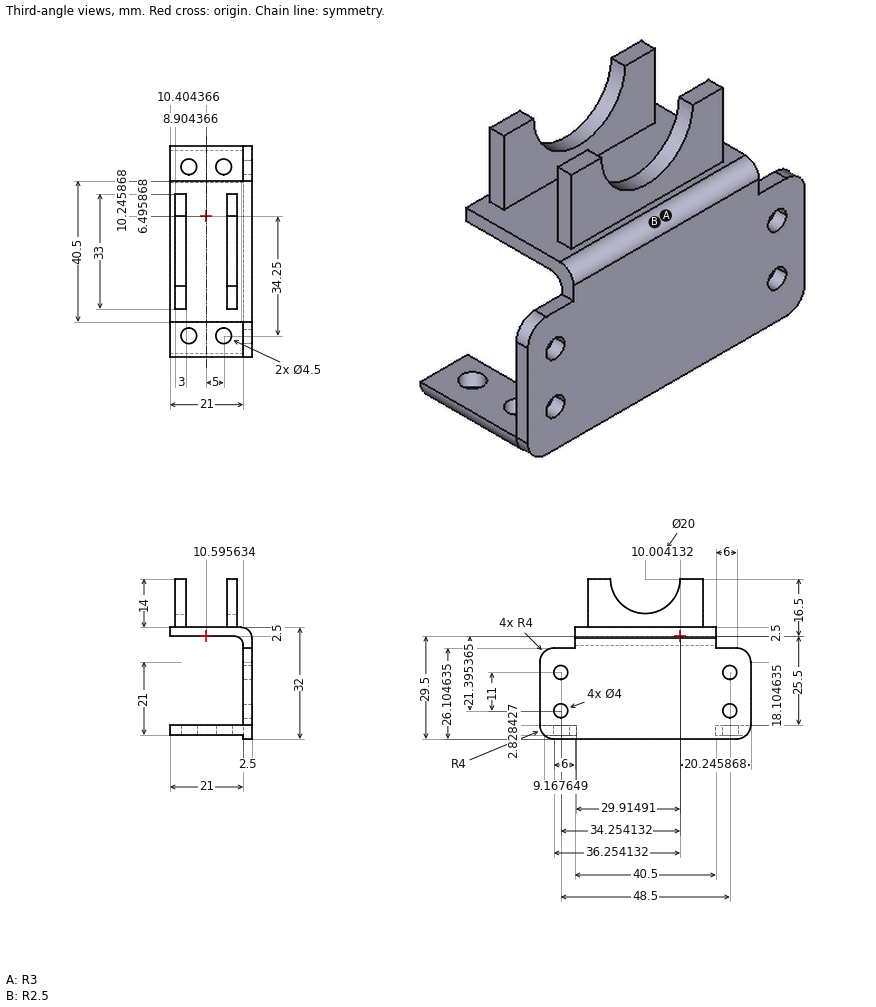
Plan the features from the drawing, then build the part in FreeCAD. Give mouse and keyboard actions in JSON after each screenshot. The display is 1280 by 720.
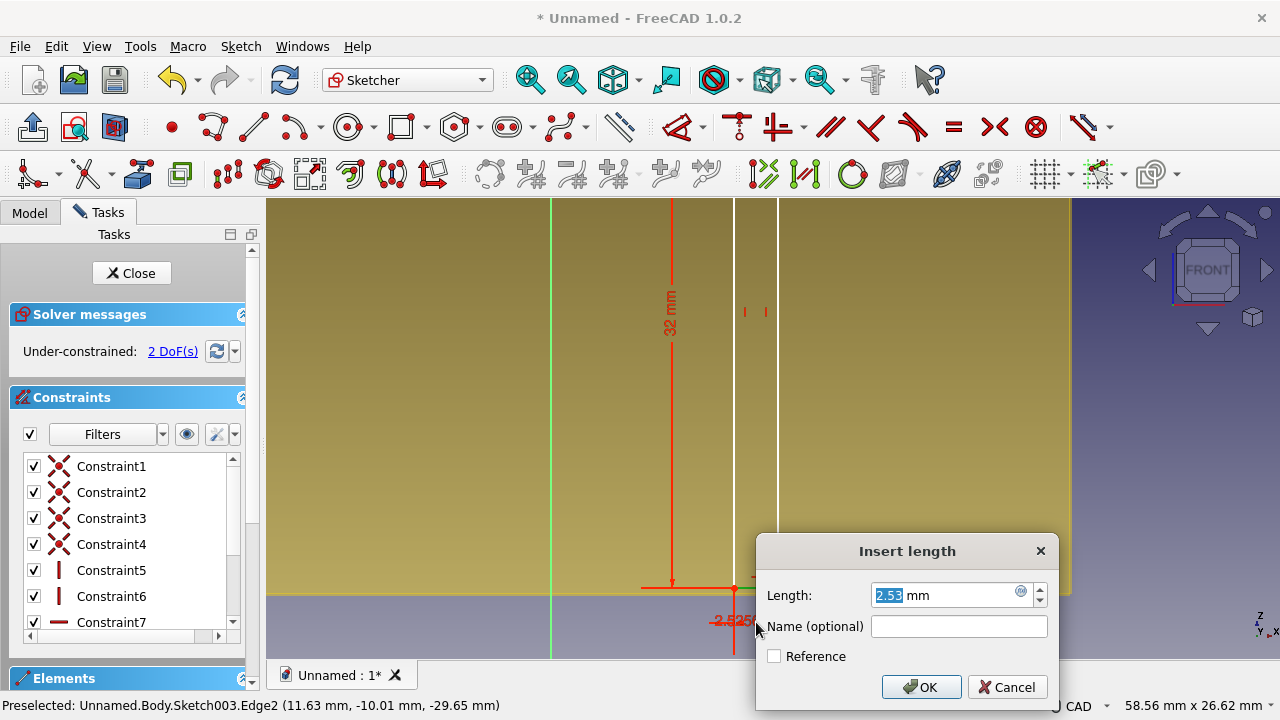
{"action": "type", "text": "2.5"}
{"action": "key", "text": "Return"}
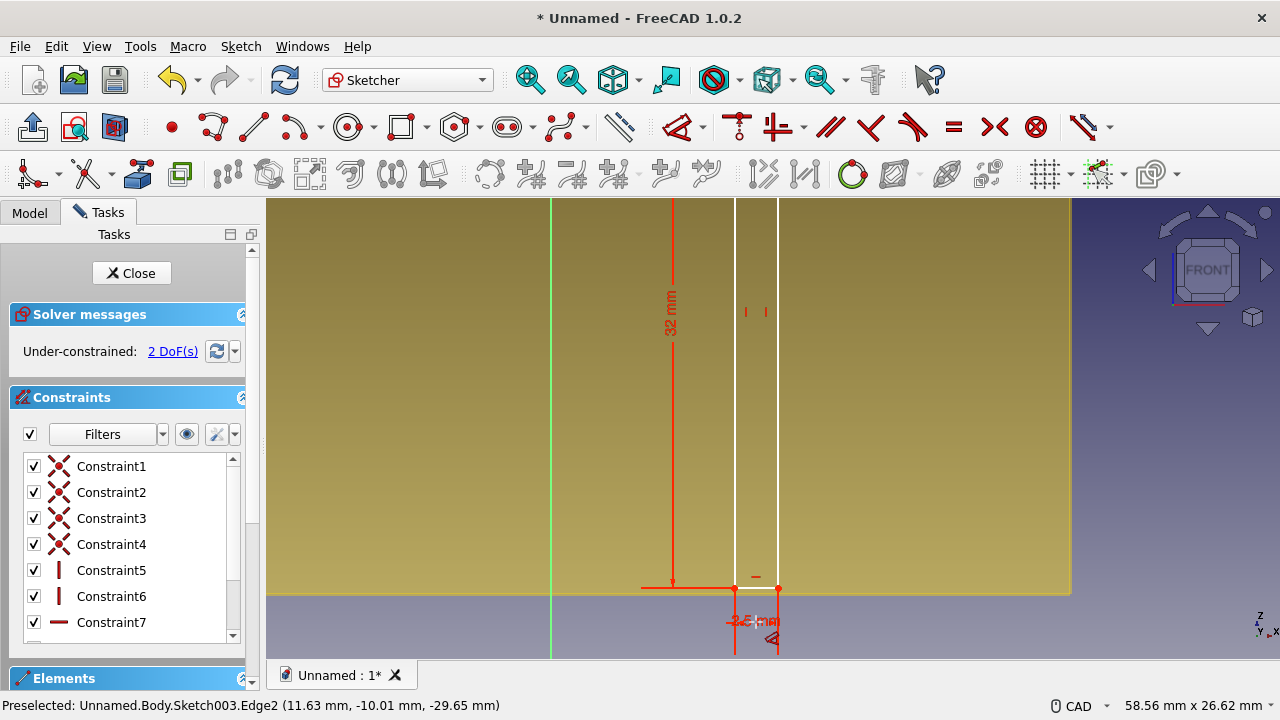
{"action": "scroll", "coordinate": [754, 574], "scroll_direction": "down", "scroll_amount": 3}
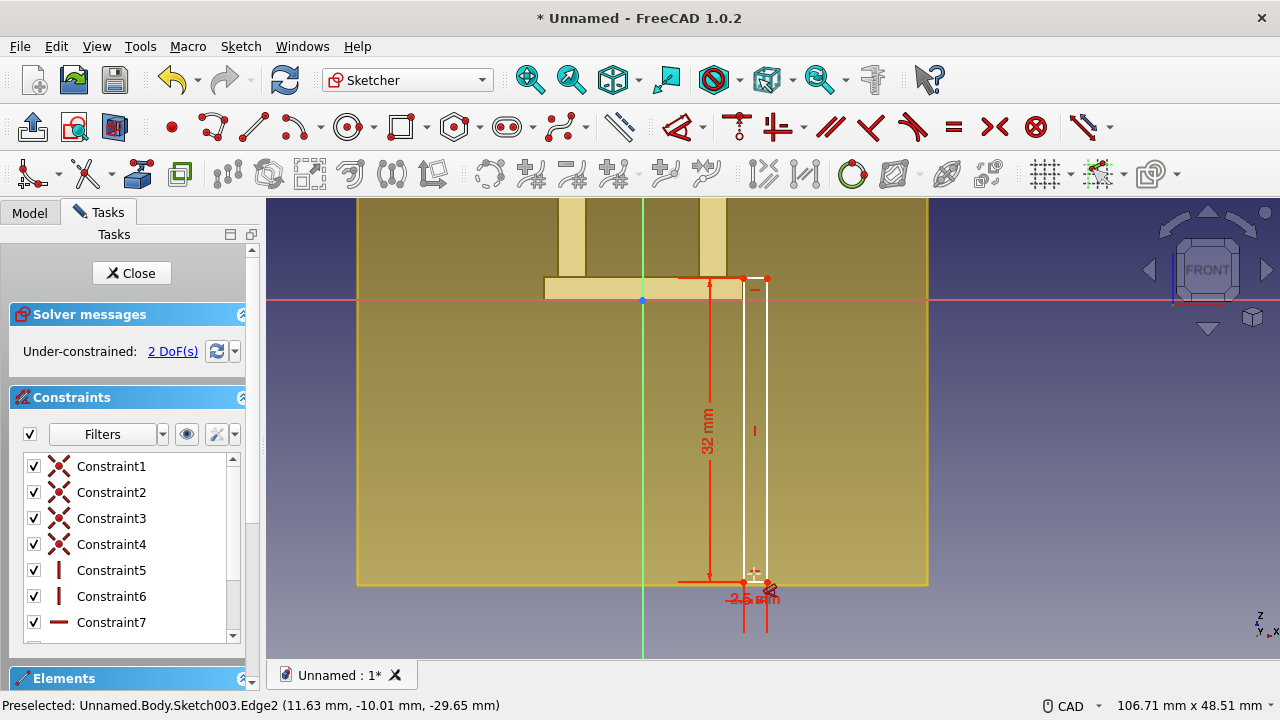
{"action": "scroll", "coordinate": [744, 278], "scroll_direction": "up", "scroll_amount": 3}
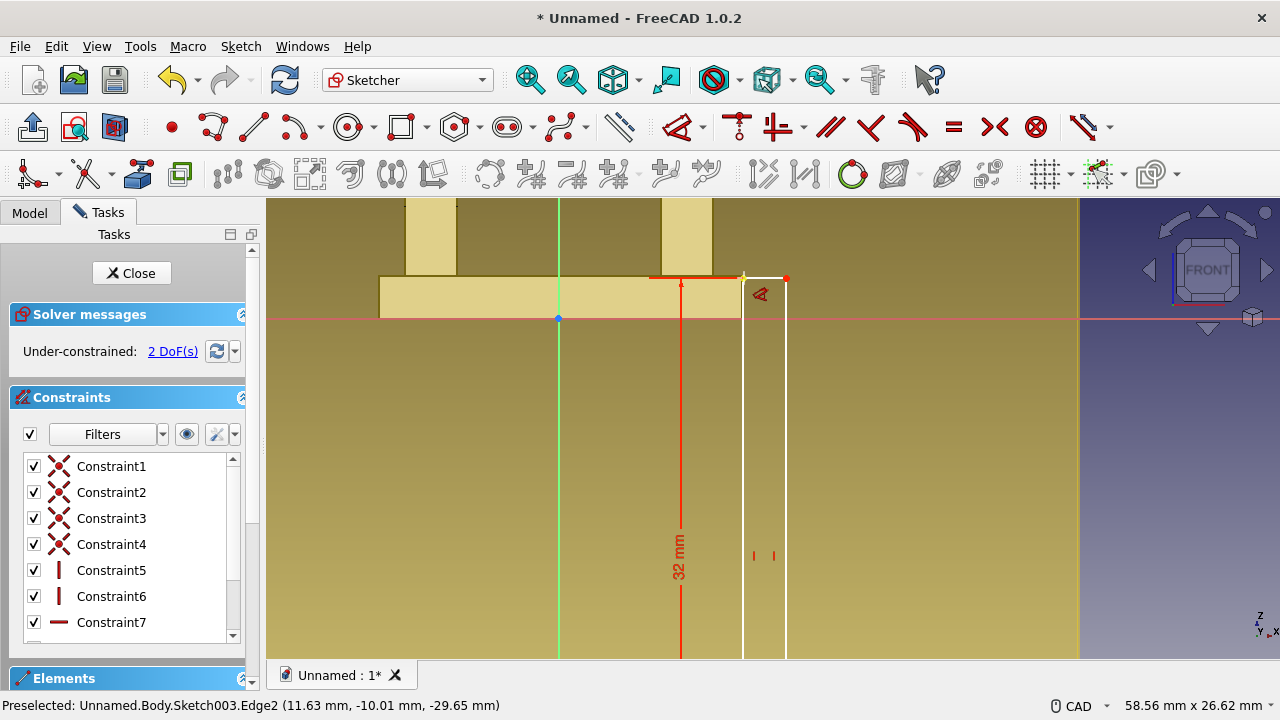
{"action": "left_click", "coordinate": [743, 278]}
{"action": "left_click", "coordinate": [525, 298]}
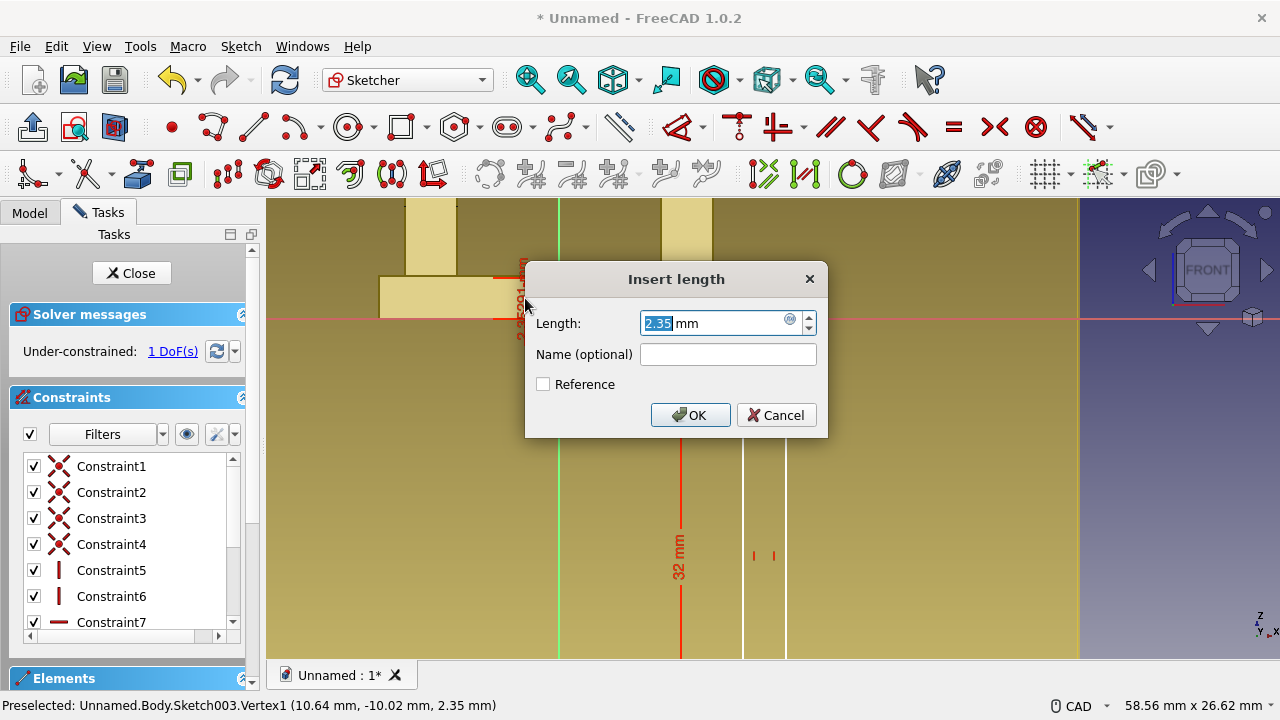
{"action": "type", "text": "2.5"}
{"action": "key", "text": "Return"}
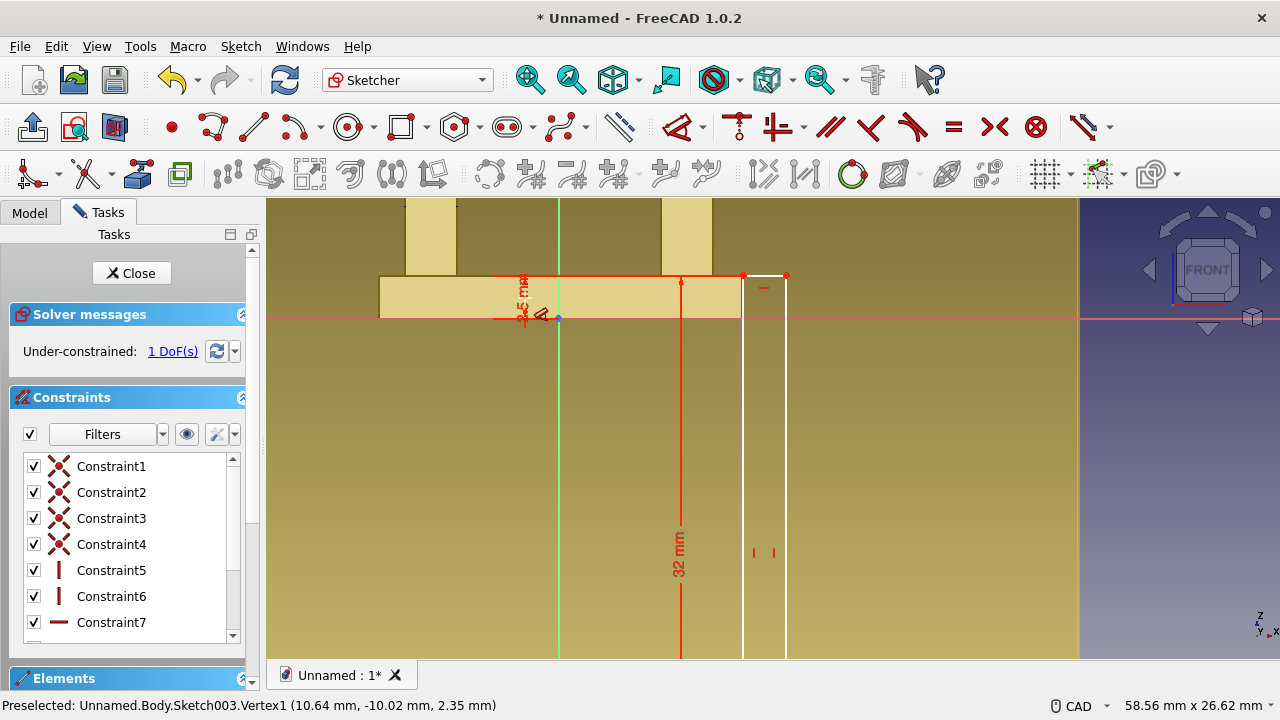
{"action": "left_click", "coordinate": [743, 276]}
{"action": "left_click", "coordinate": [651, 242]}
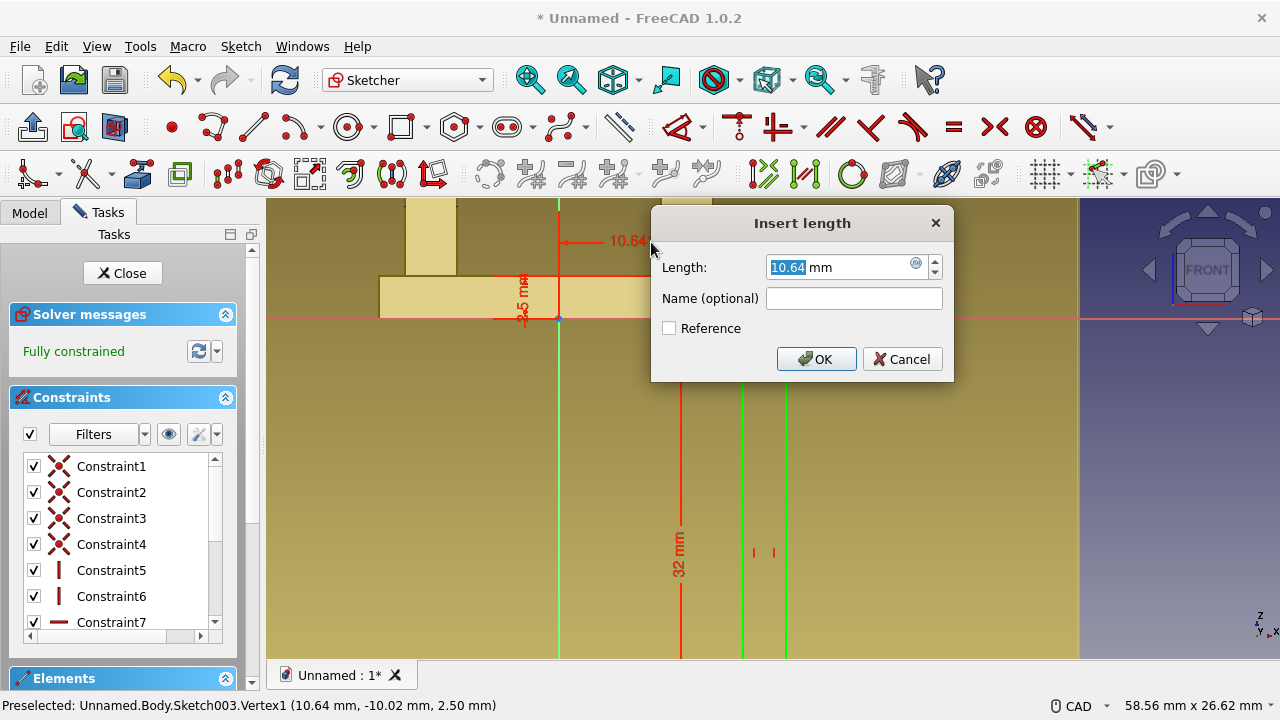
{"action": "type", "text": "10.595634"}
{"action": "key", "text": "Return"}
{"action": "key", "text": "Escape"}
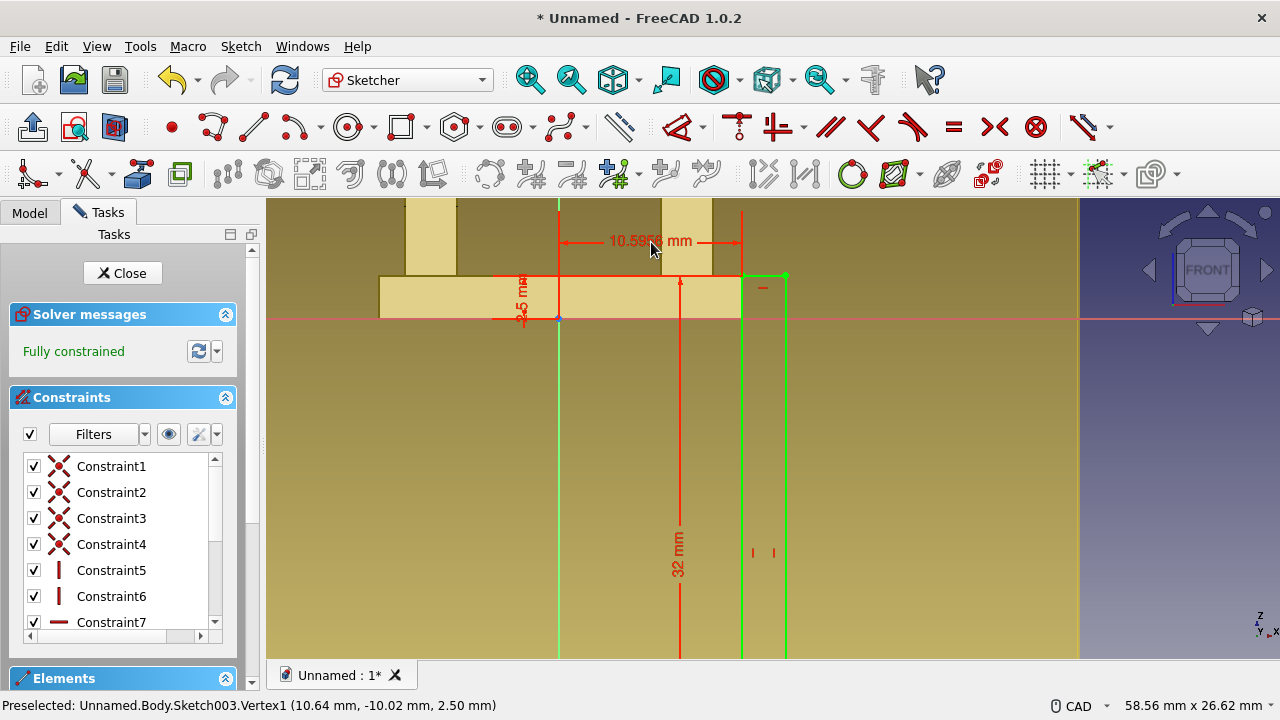
{"action": "left_click", "coordinate": [123, 273]}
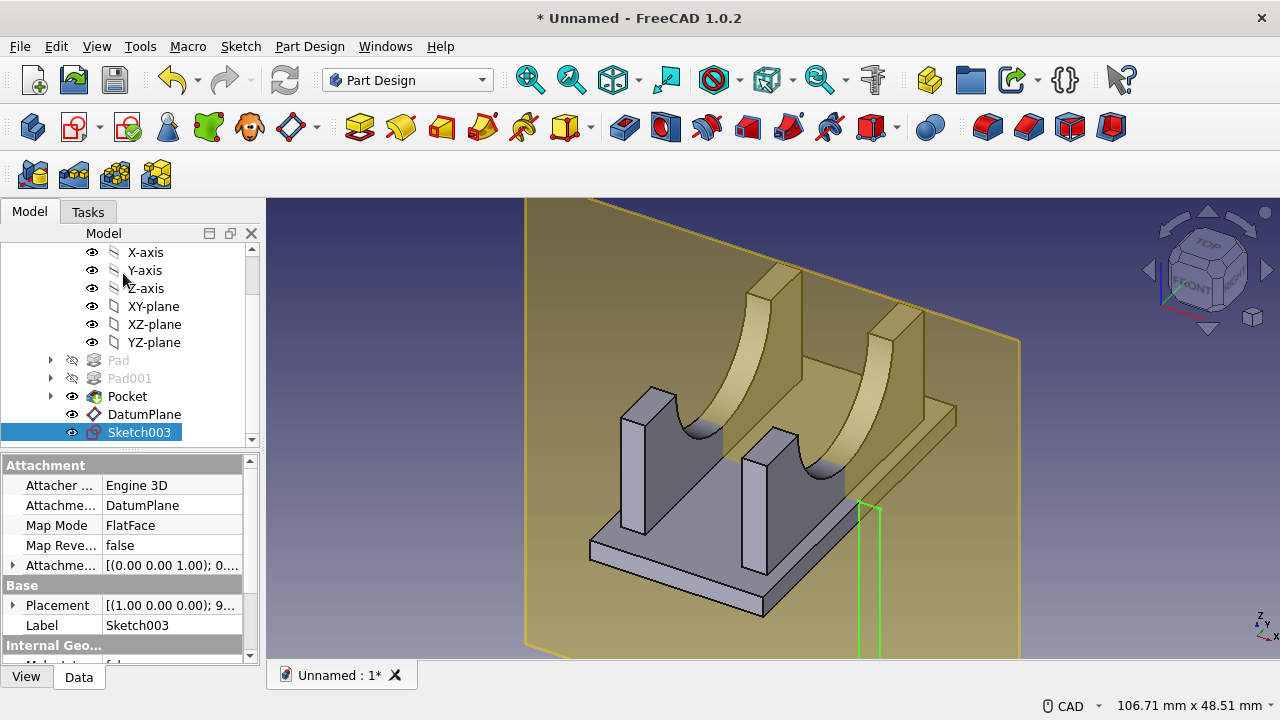
{"action": "left_click", "coordinate": [360, 128]}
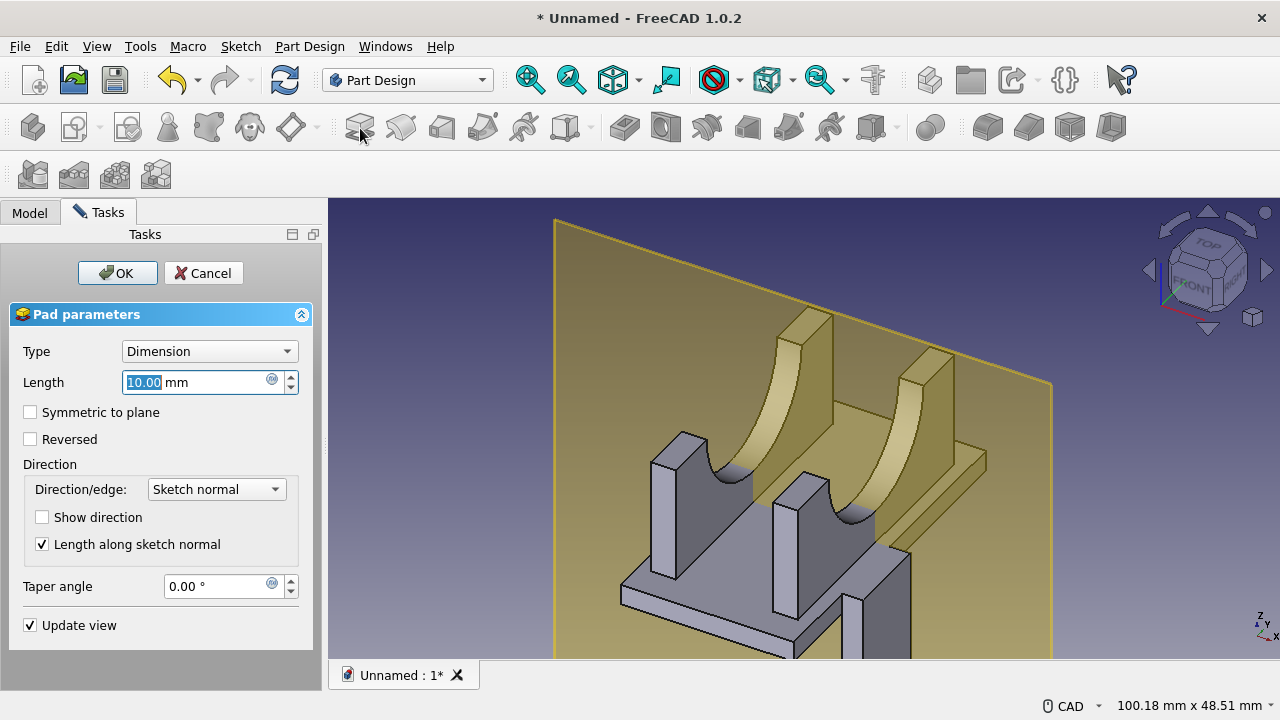
{"action": "type", "text": "40.5"}
{"action": "key", "text": "Tab"}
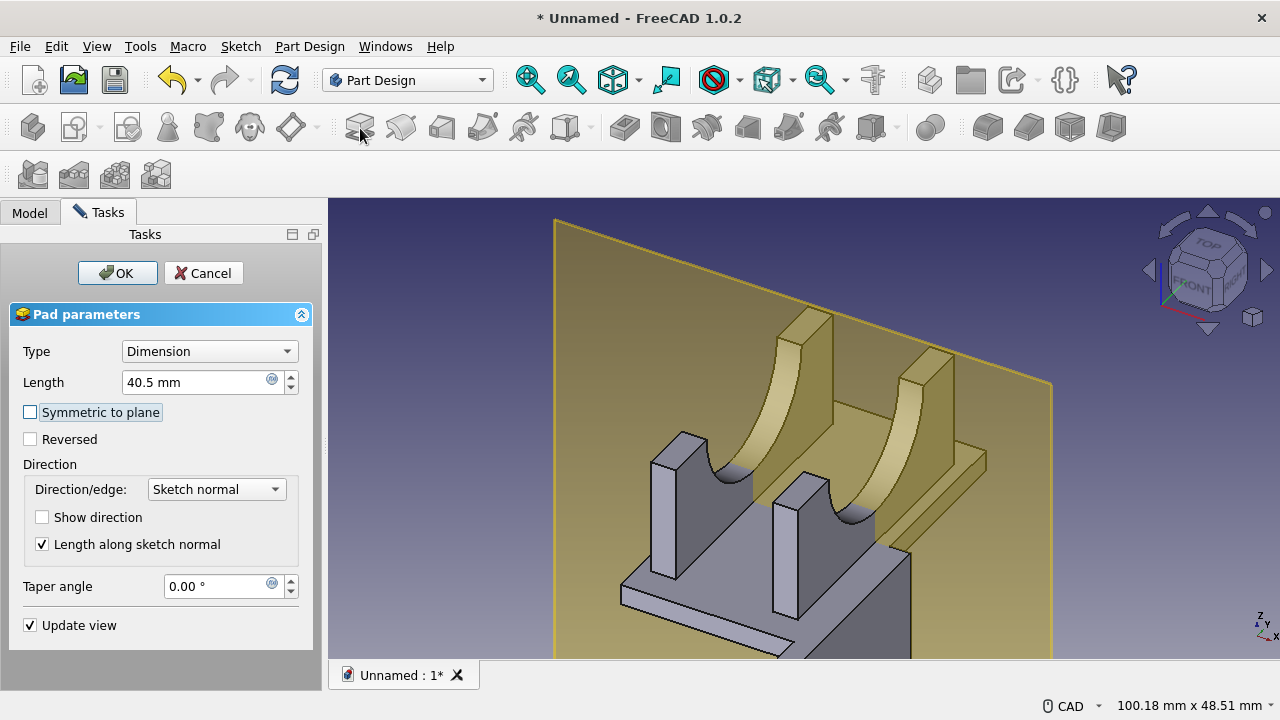
{"action": "left_click", "coordinate": [31, 412]}